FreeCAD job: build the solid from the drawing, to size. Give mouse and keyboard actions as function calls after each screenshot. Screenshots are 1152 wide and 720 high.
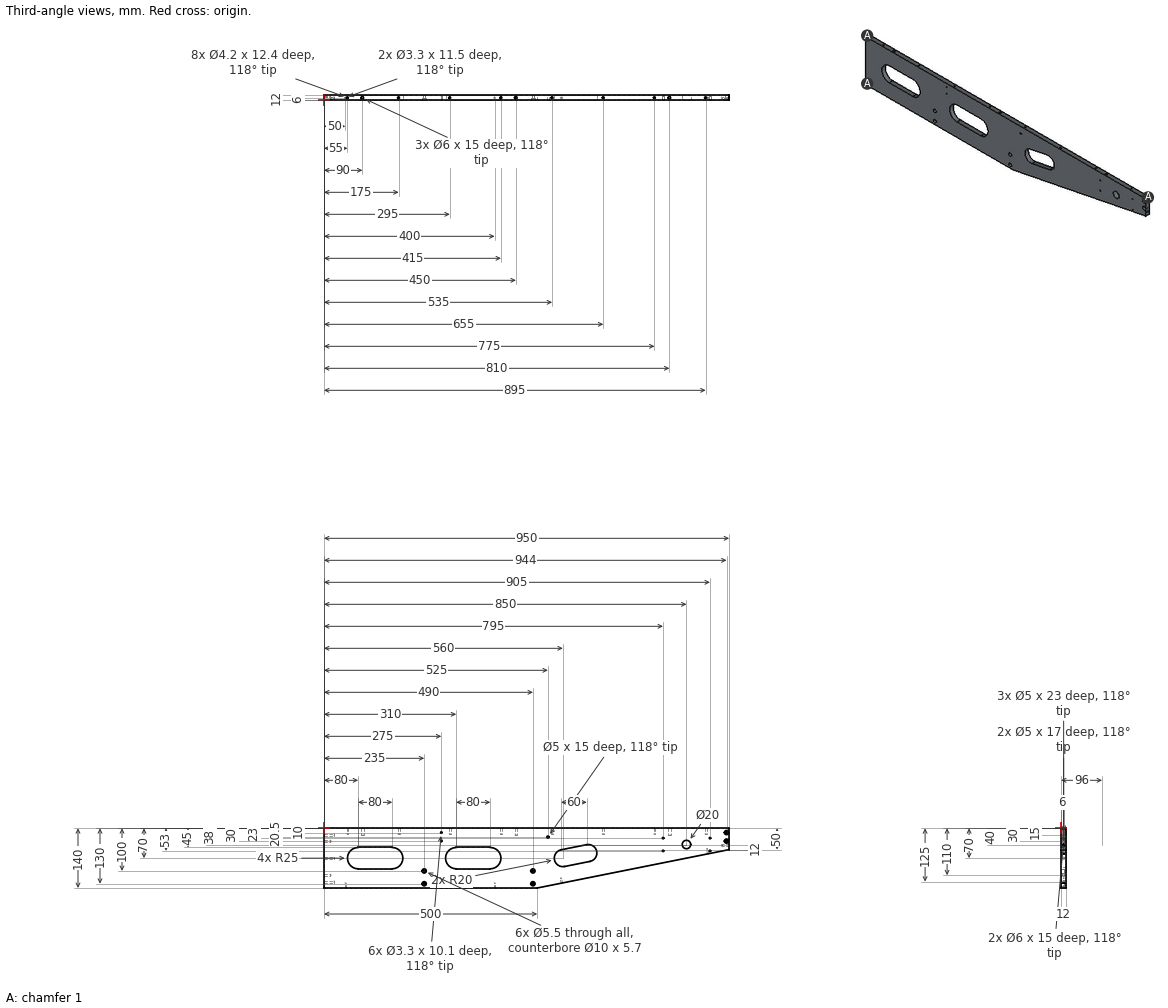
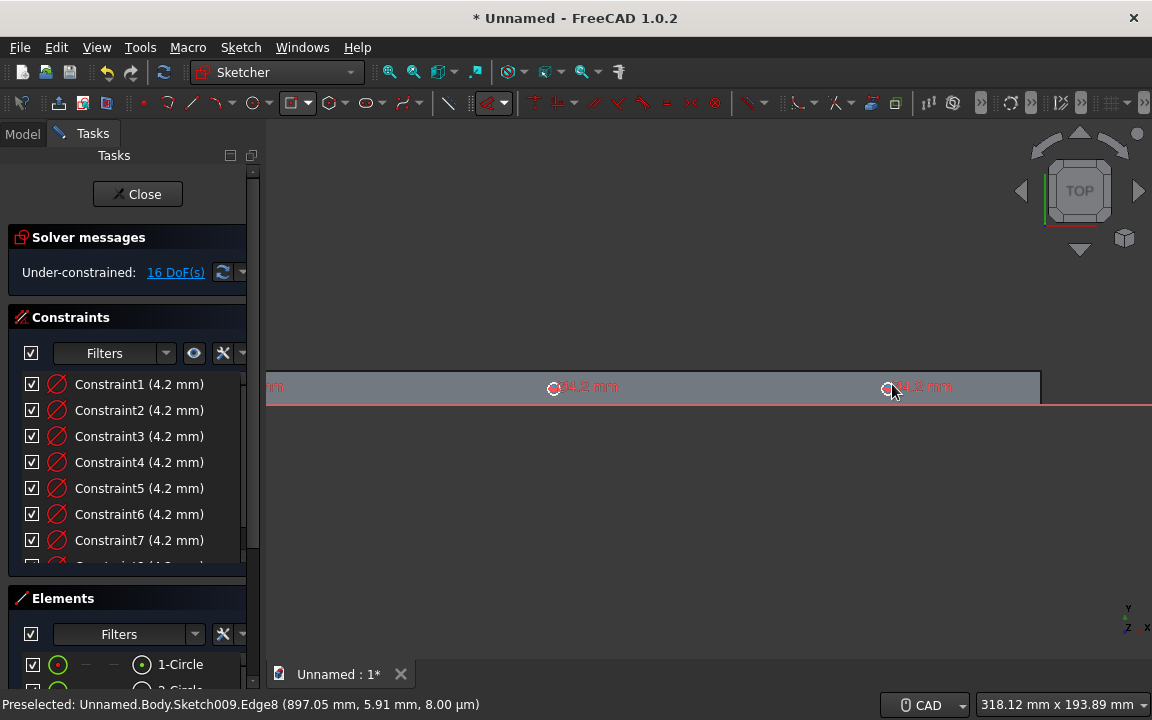
scroll(892, 388, down, 8)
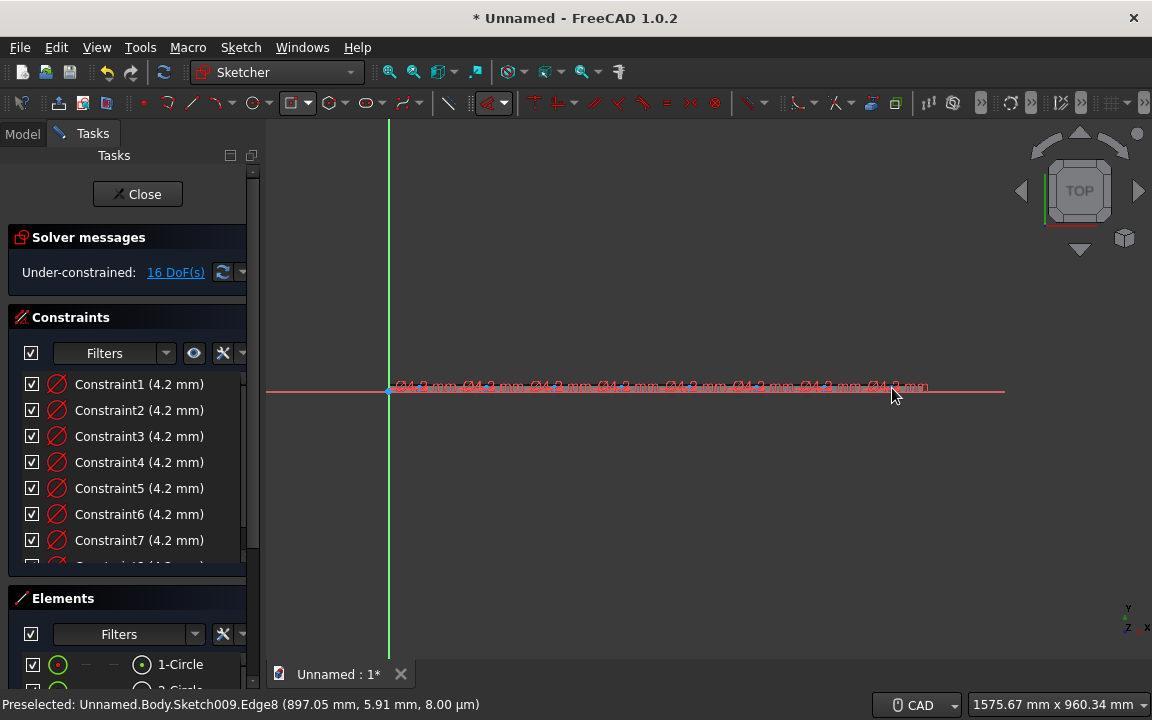
click(420, 389)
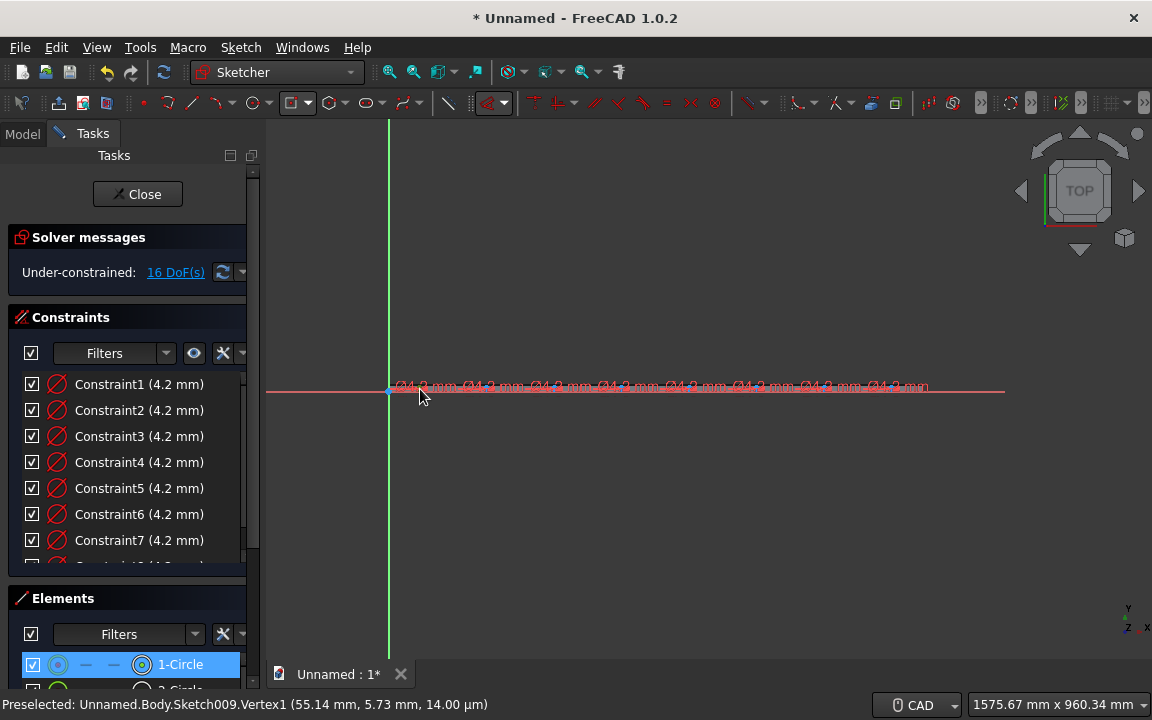
click(487, 389)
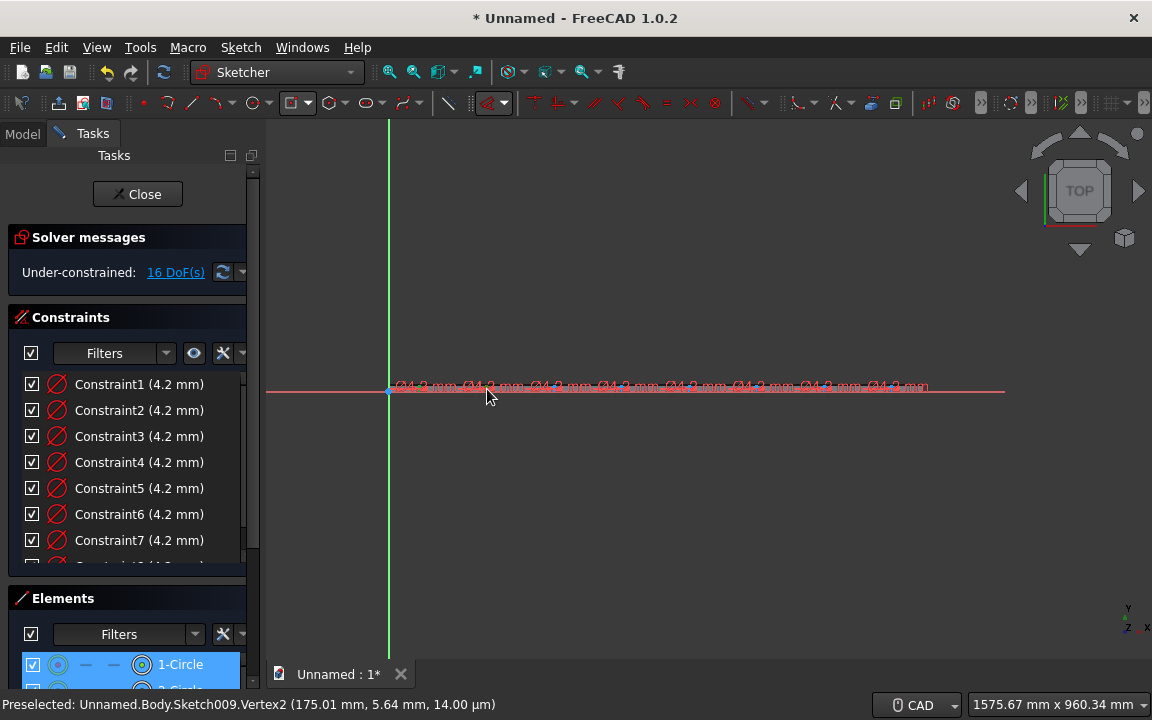
key(h)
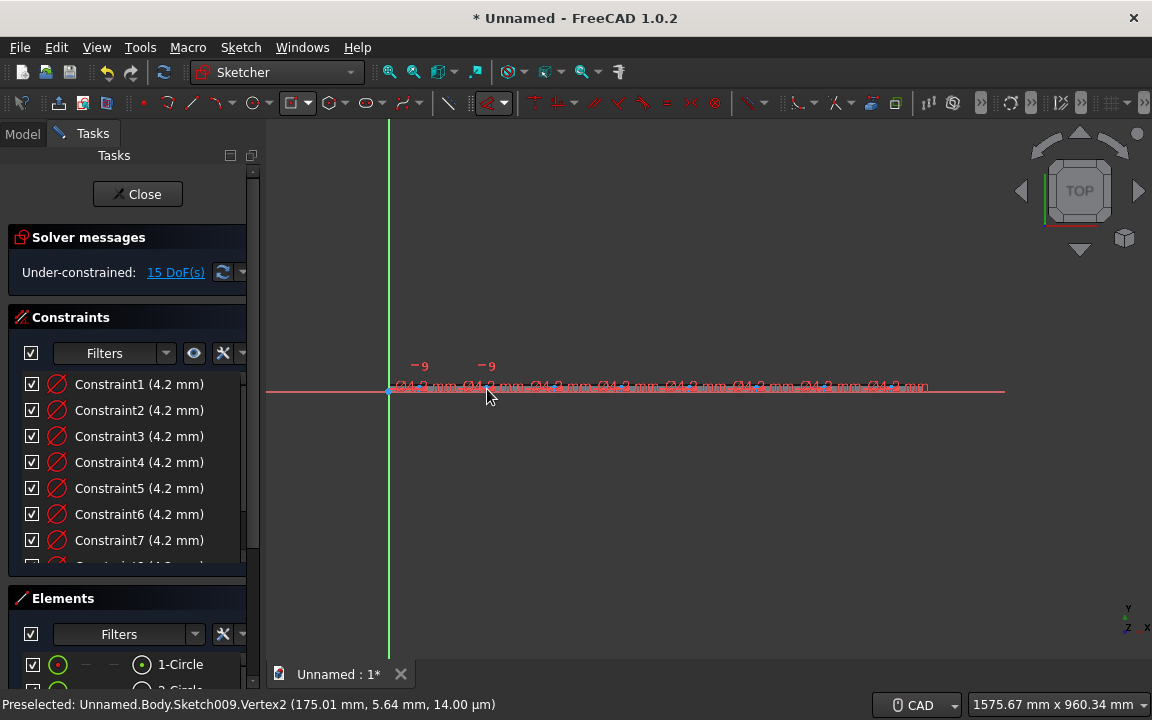
click(487, 389)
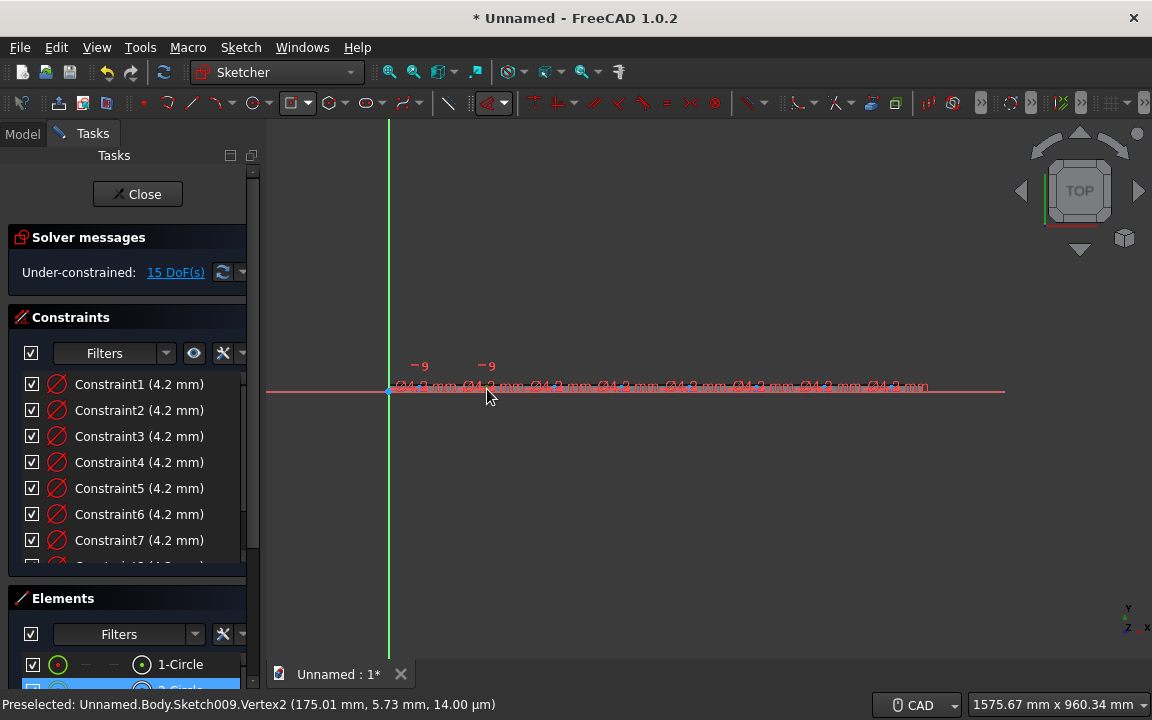
click(554, 389)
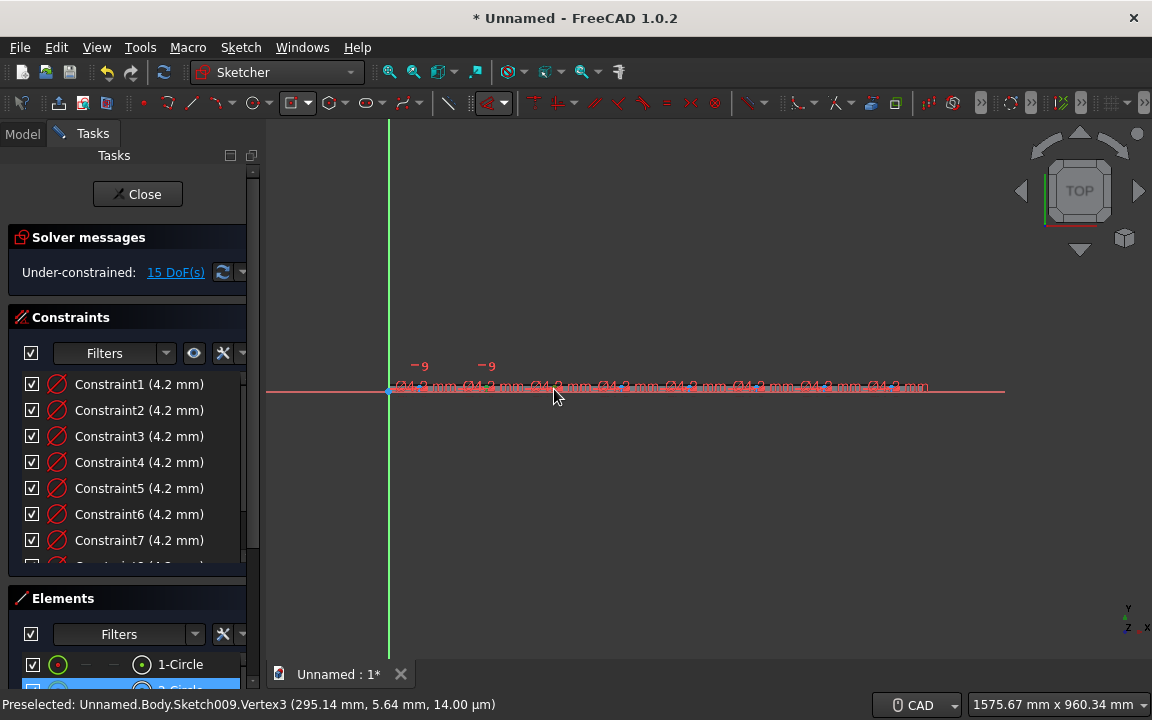
key(h)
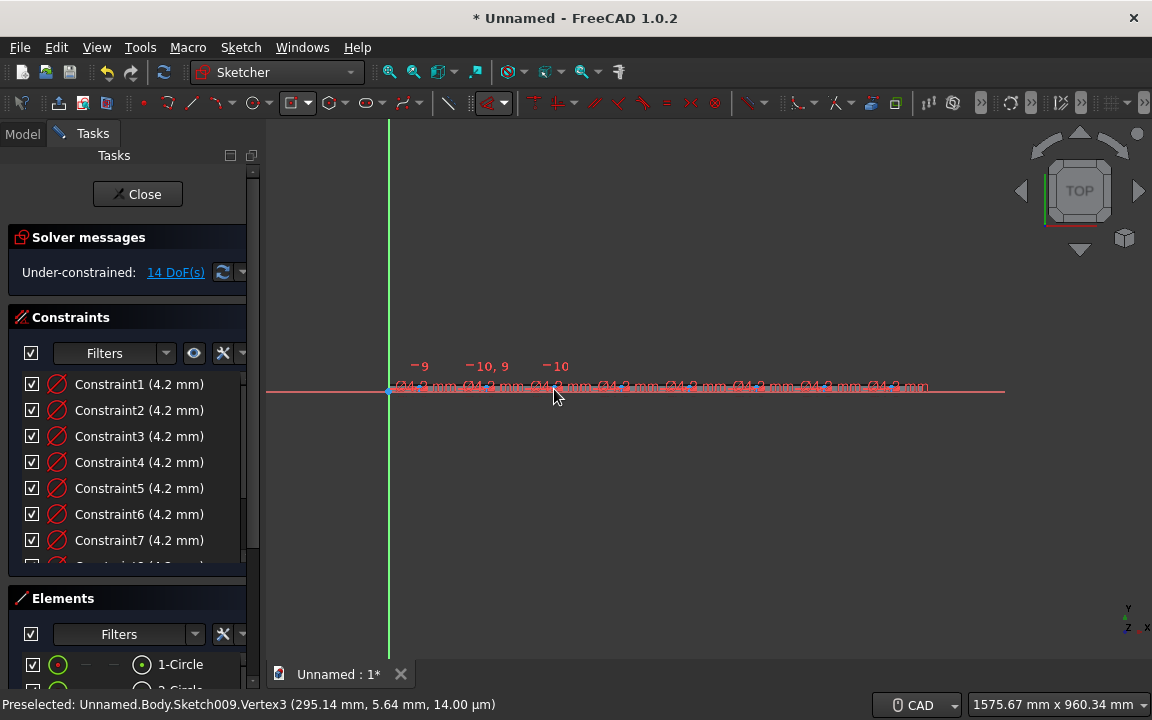
click(554, 389)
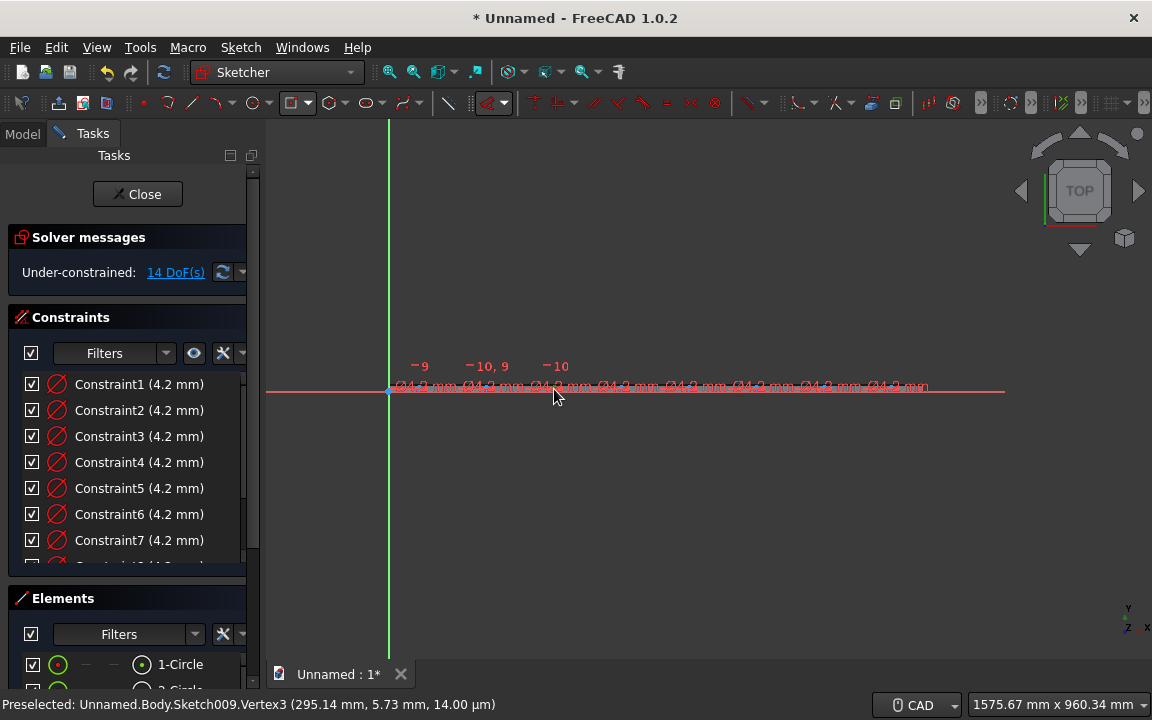
click(622, 389)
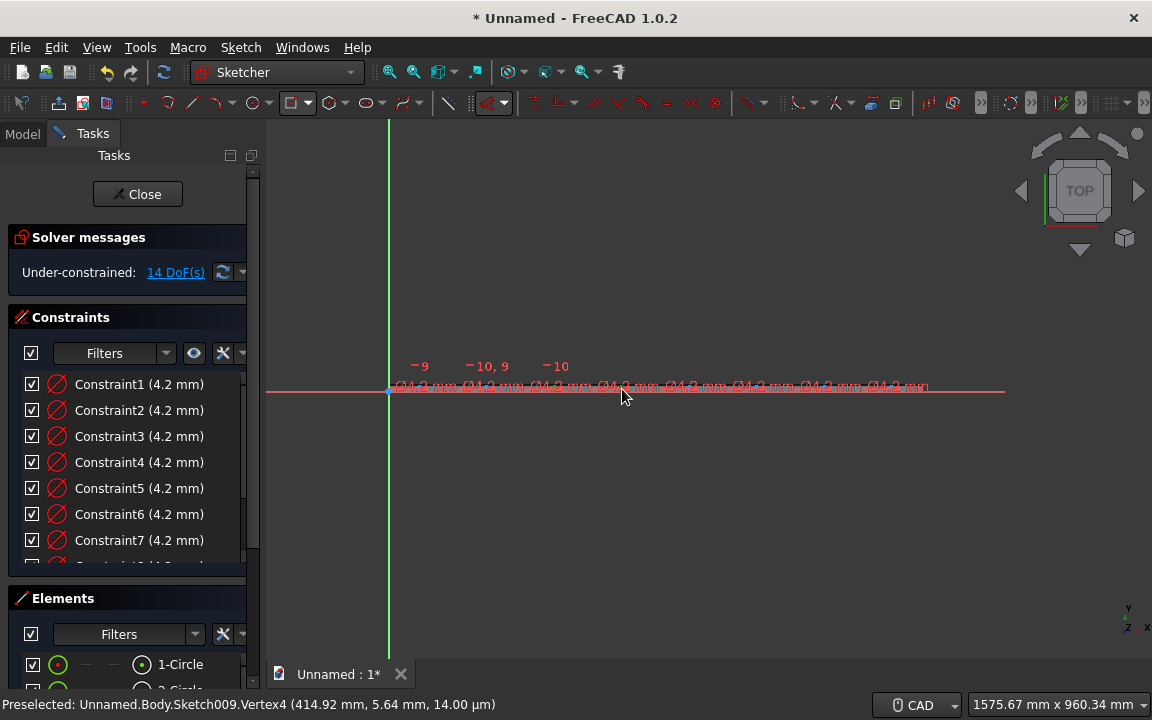
key(h)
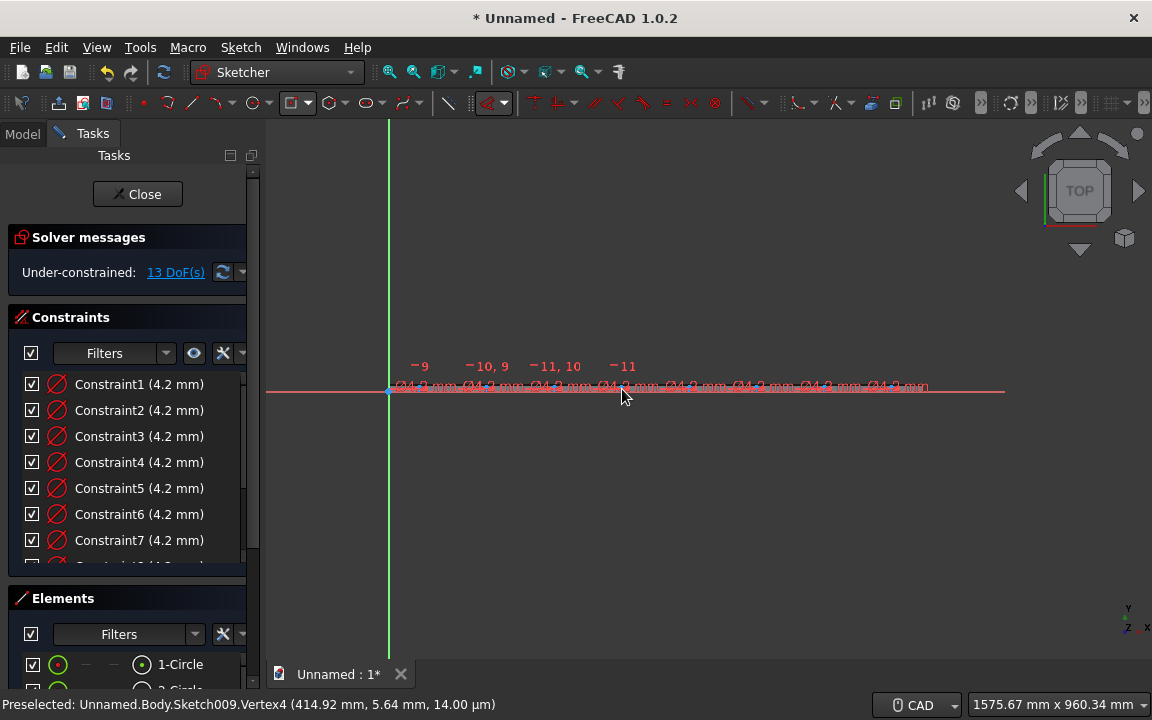
click(622, 389)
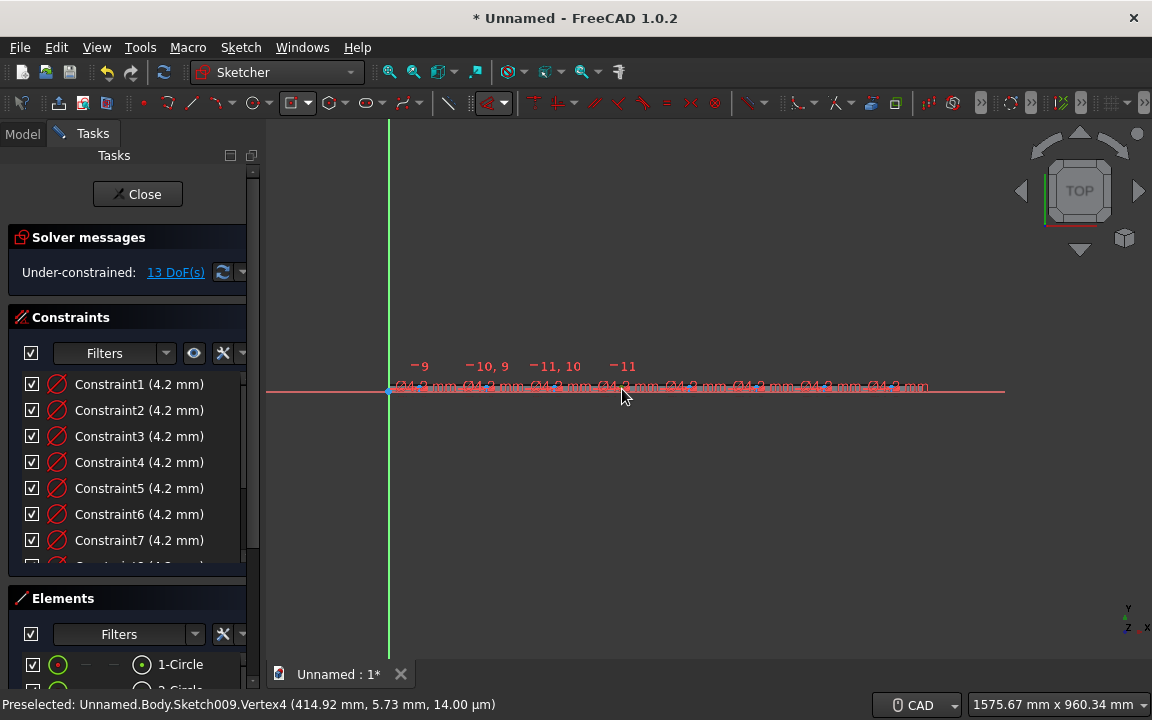
click(689, 389)